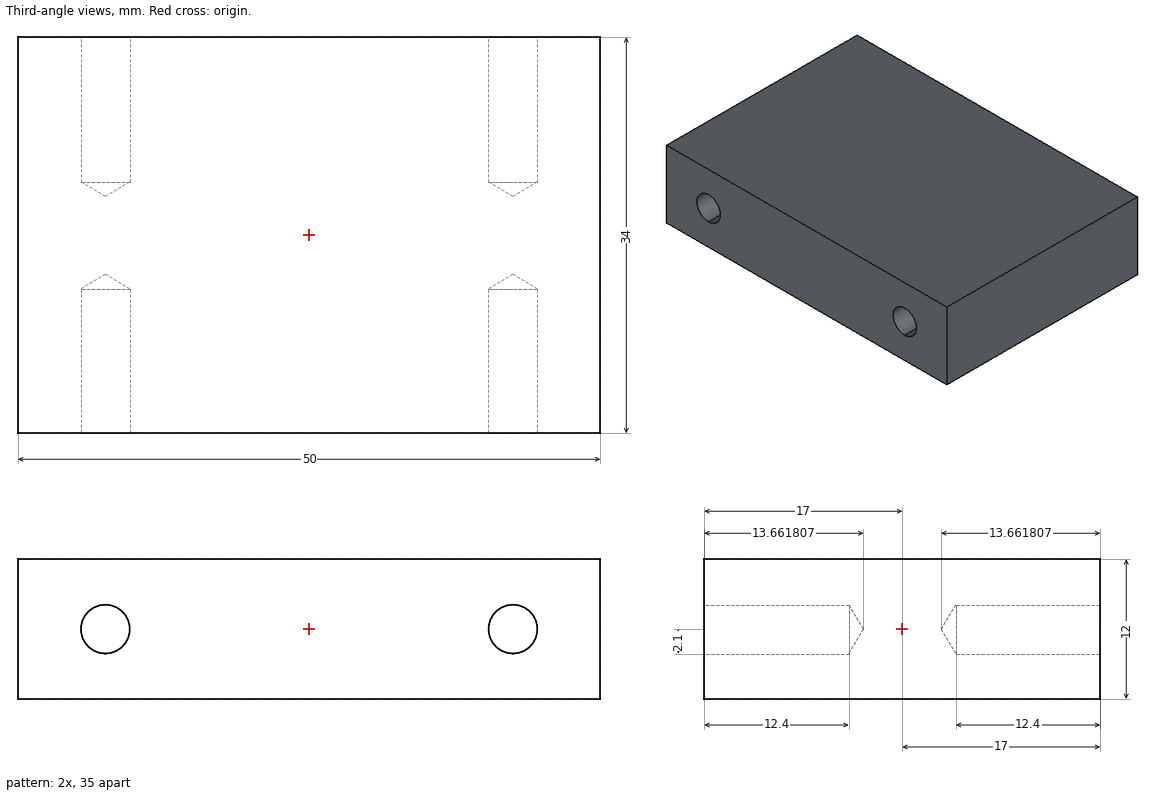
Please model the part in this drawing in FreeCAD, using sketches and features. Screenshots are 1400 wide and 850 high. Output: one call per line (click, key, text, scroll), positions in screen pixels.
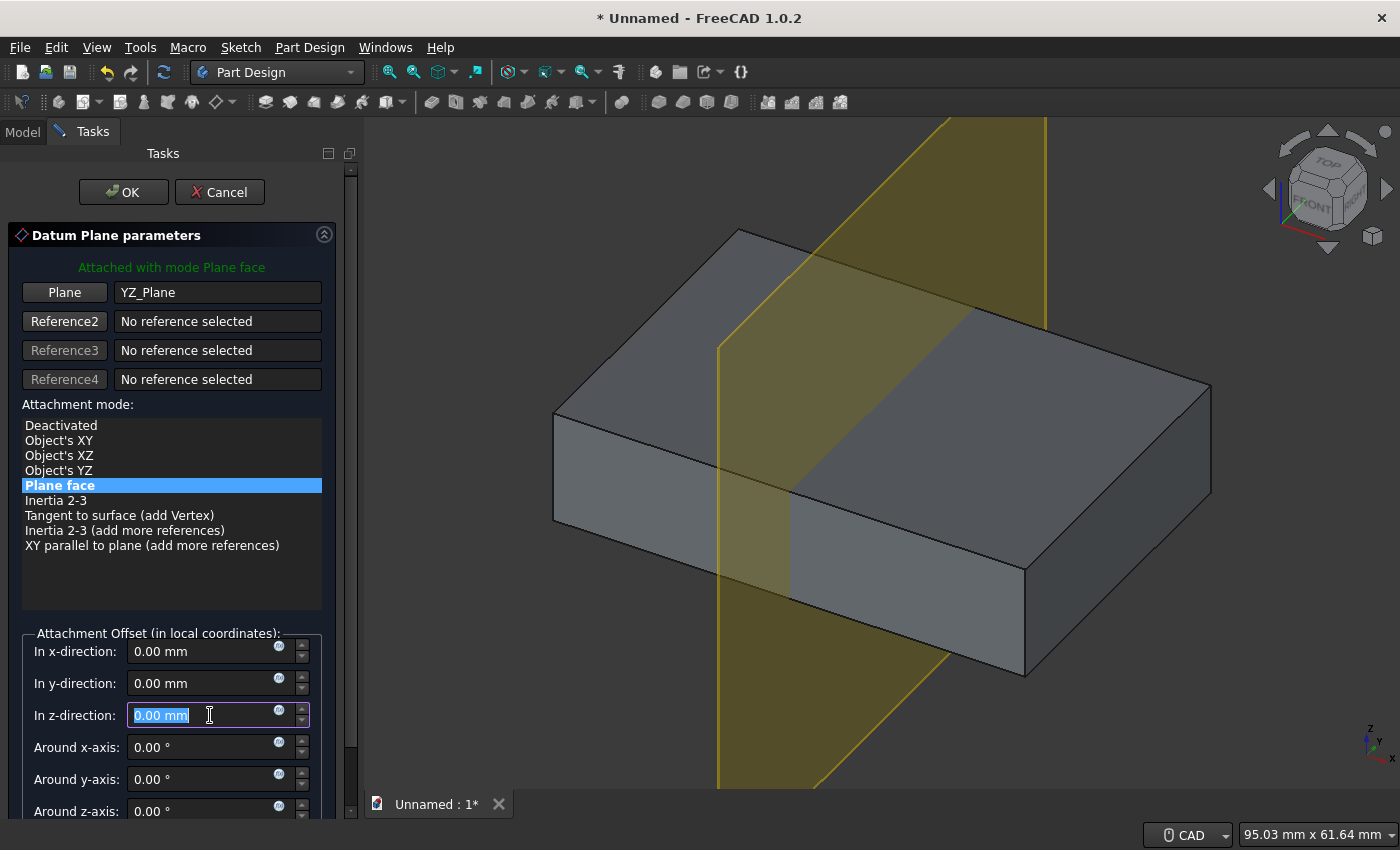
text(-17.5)
key(Tab)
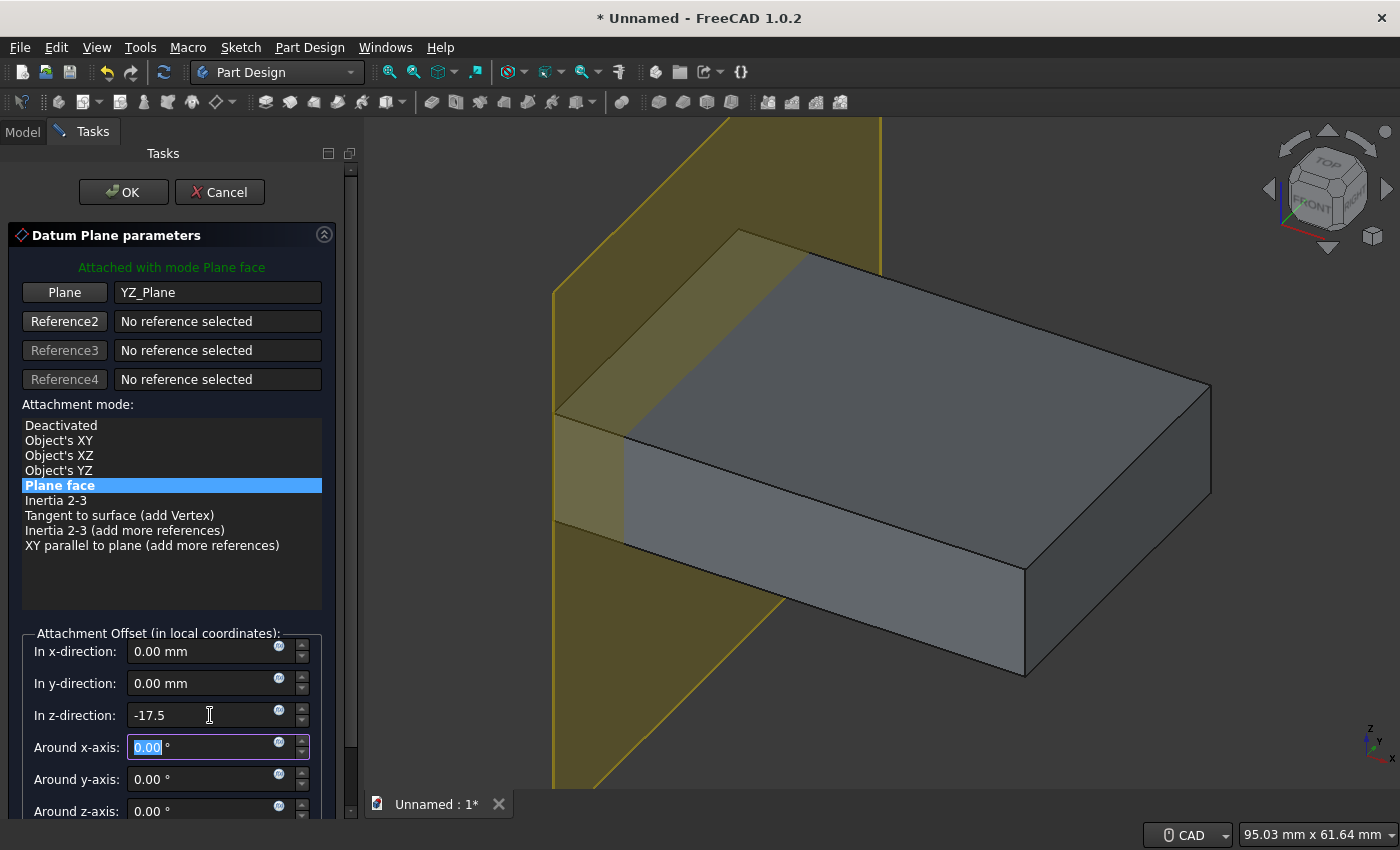
click(124, 192)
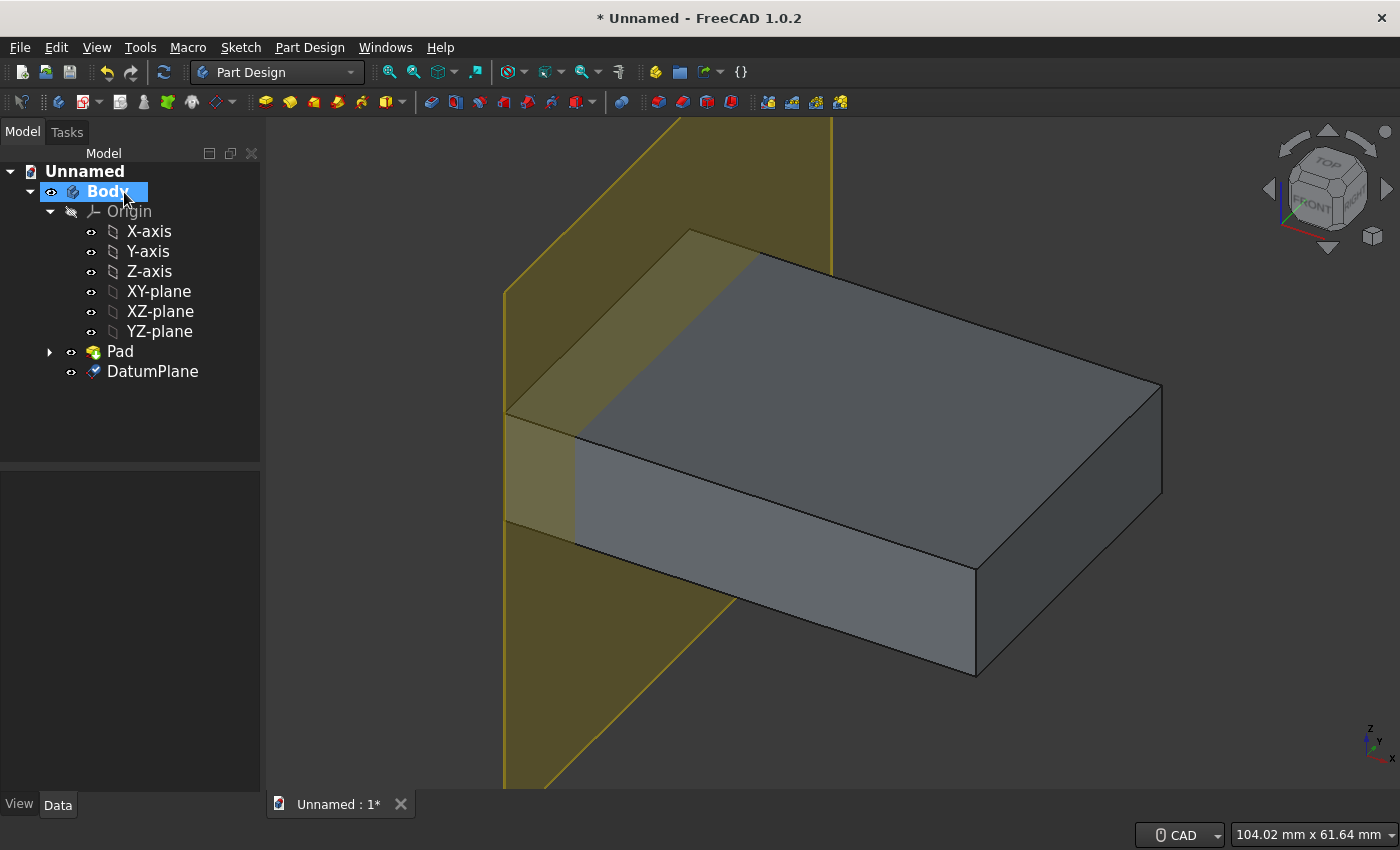
click(116, 372)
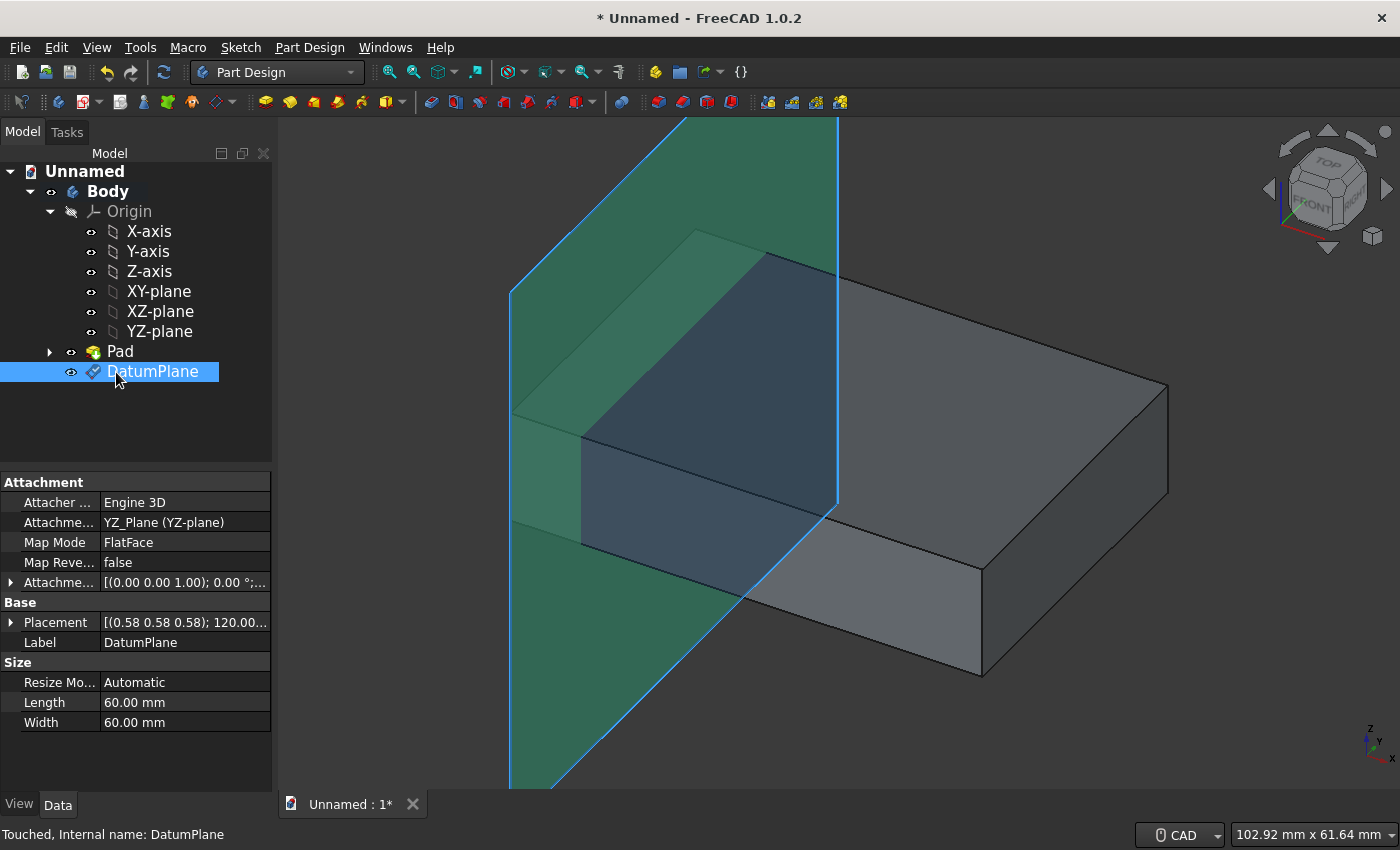
click(84, 102)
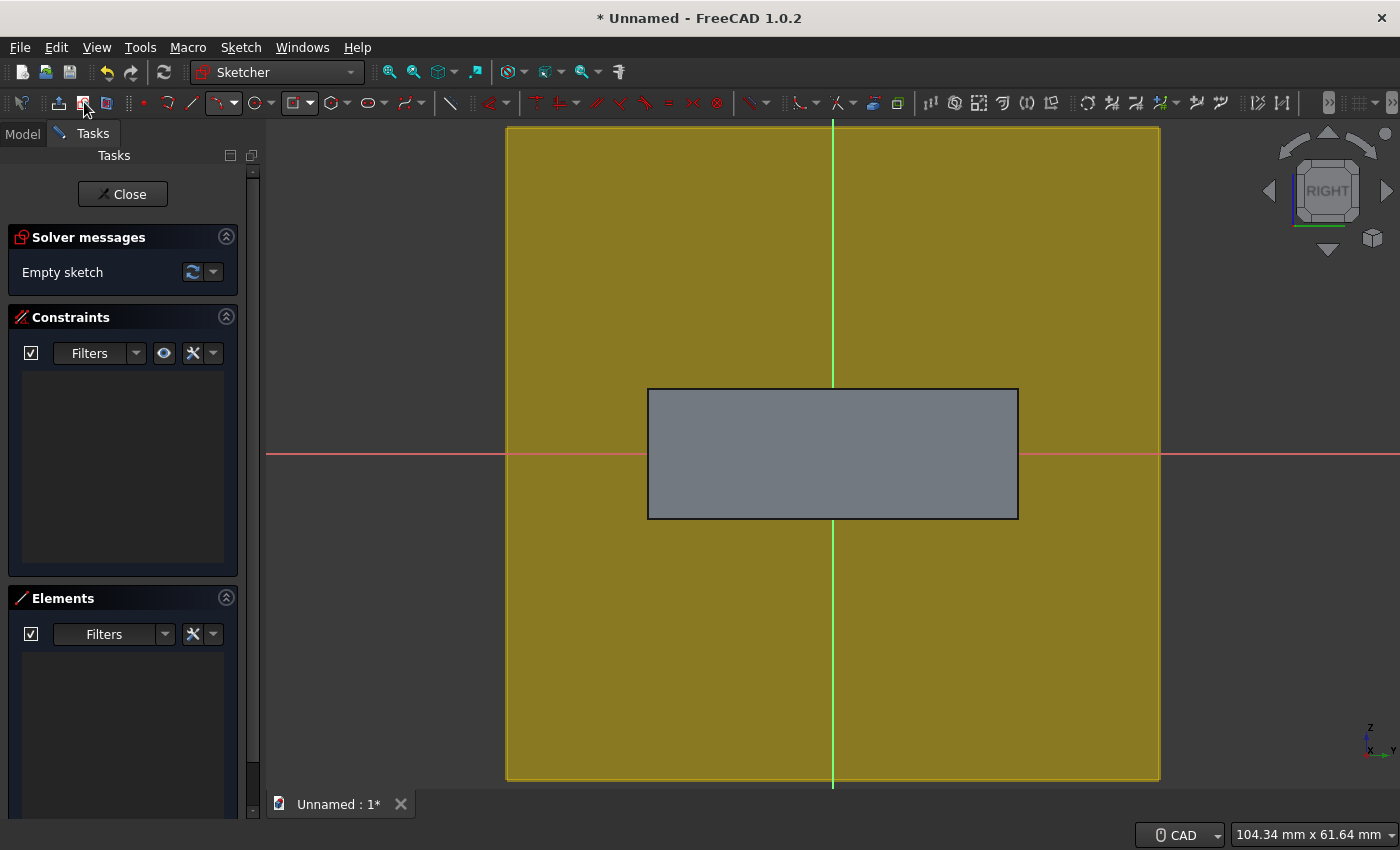
click(108, 104)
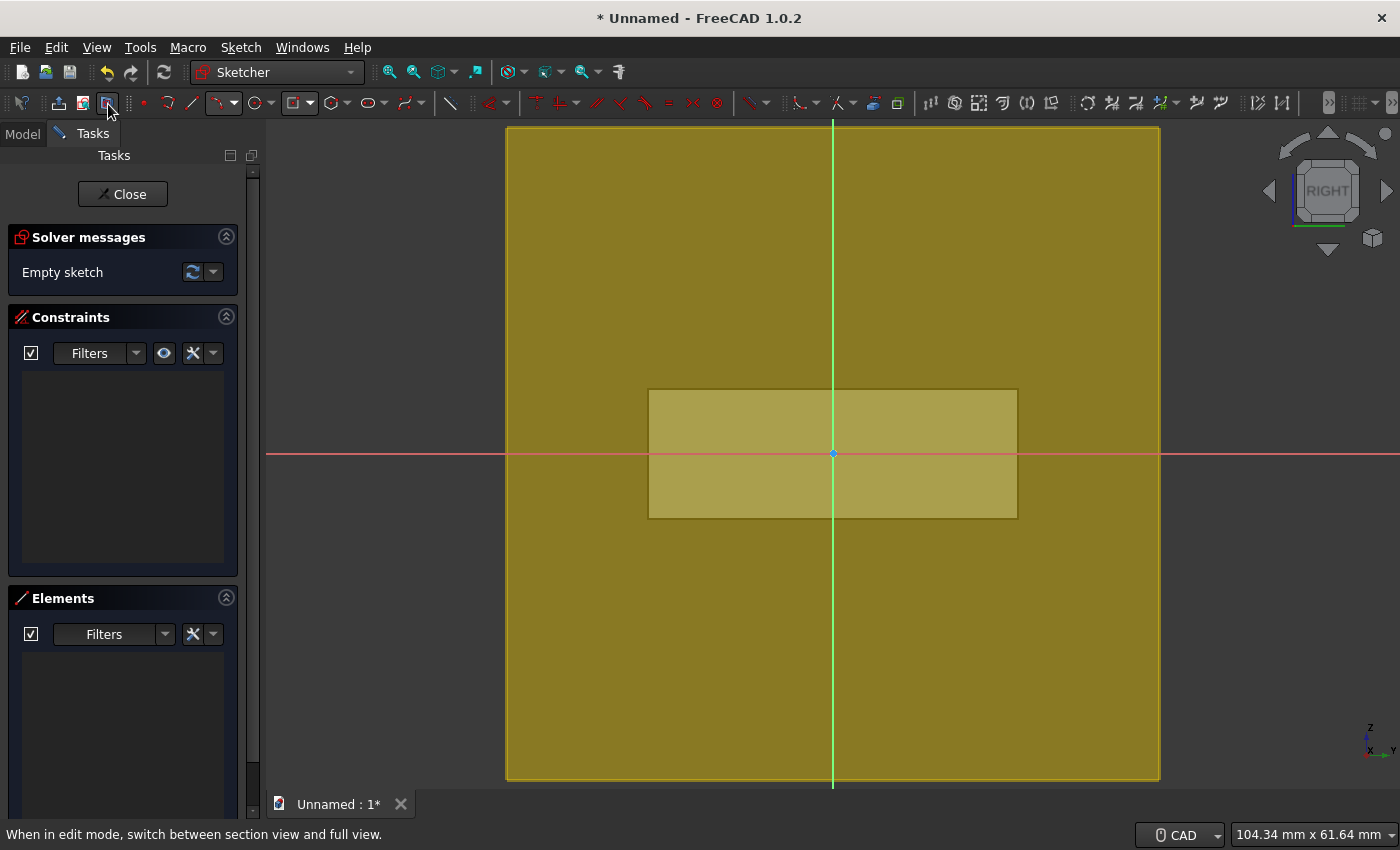
scroll(730, 470, up, 6)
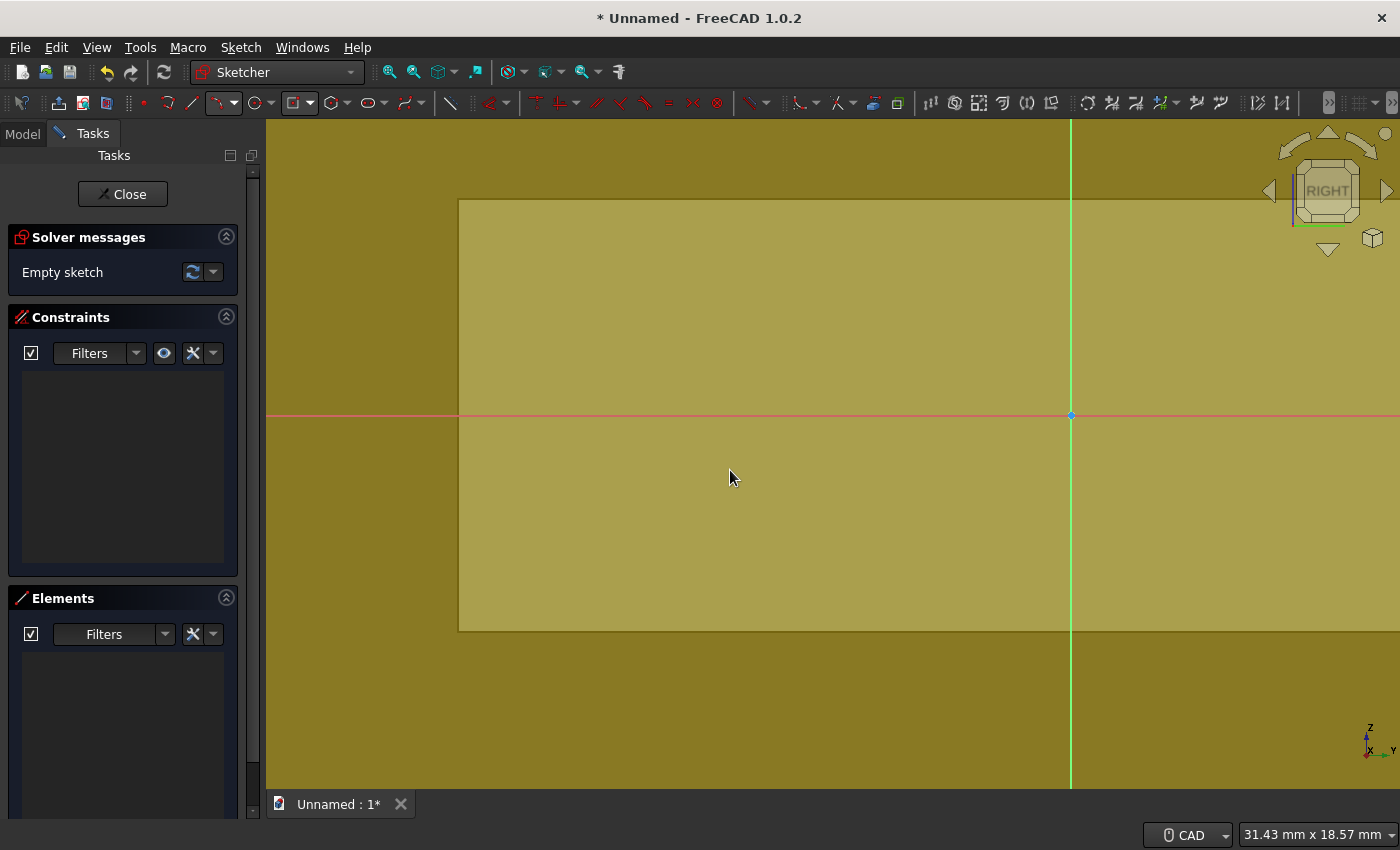
key(g)
key(m)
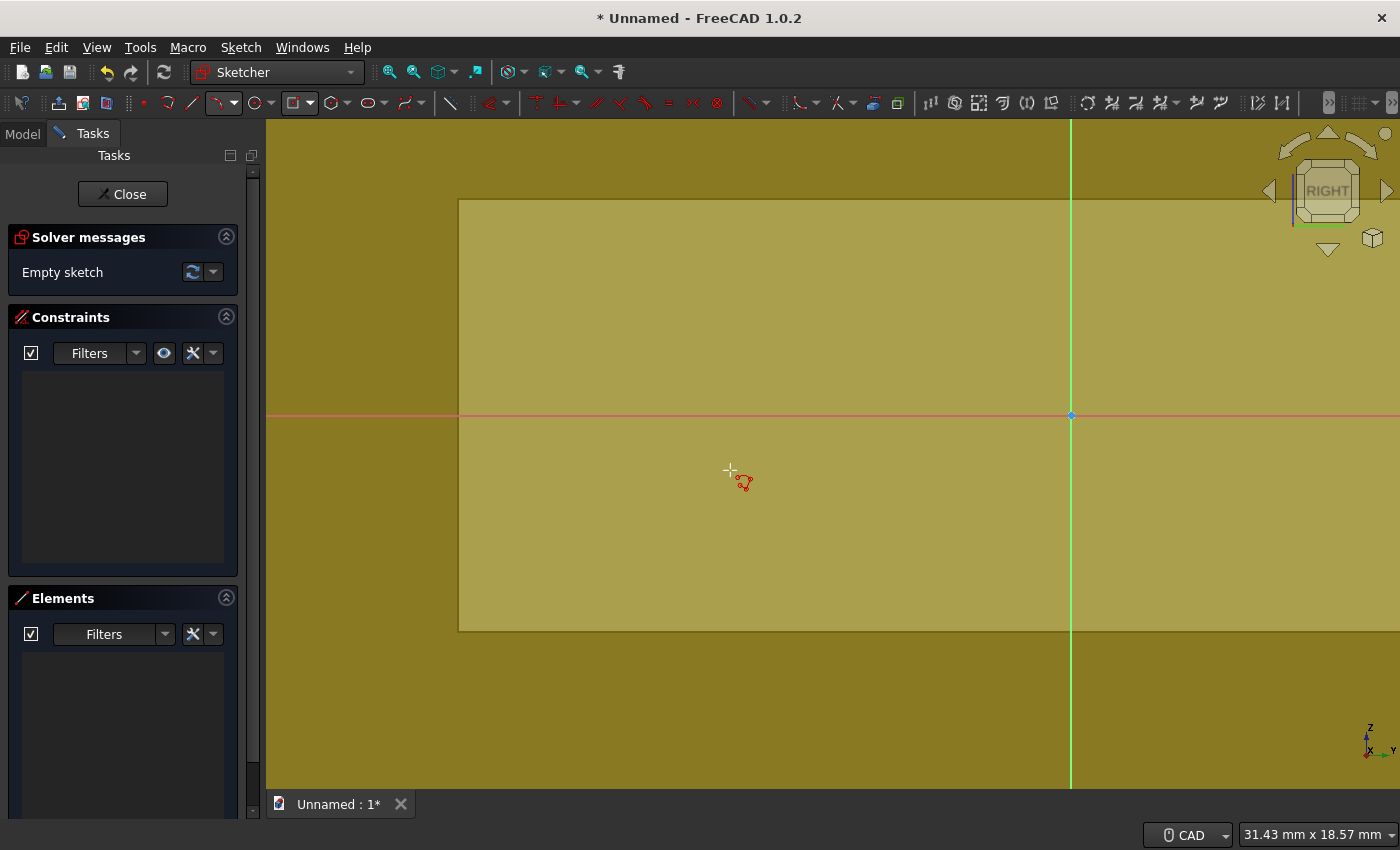
click(951, 416)
click(458, 425)
click(458, 491)
click(905, 491)
click(951, 416)
key(Escape)
key(Escape)